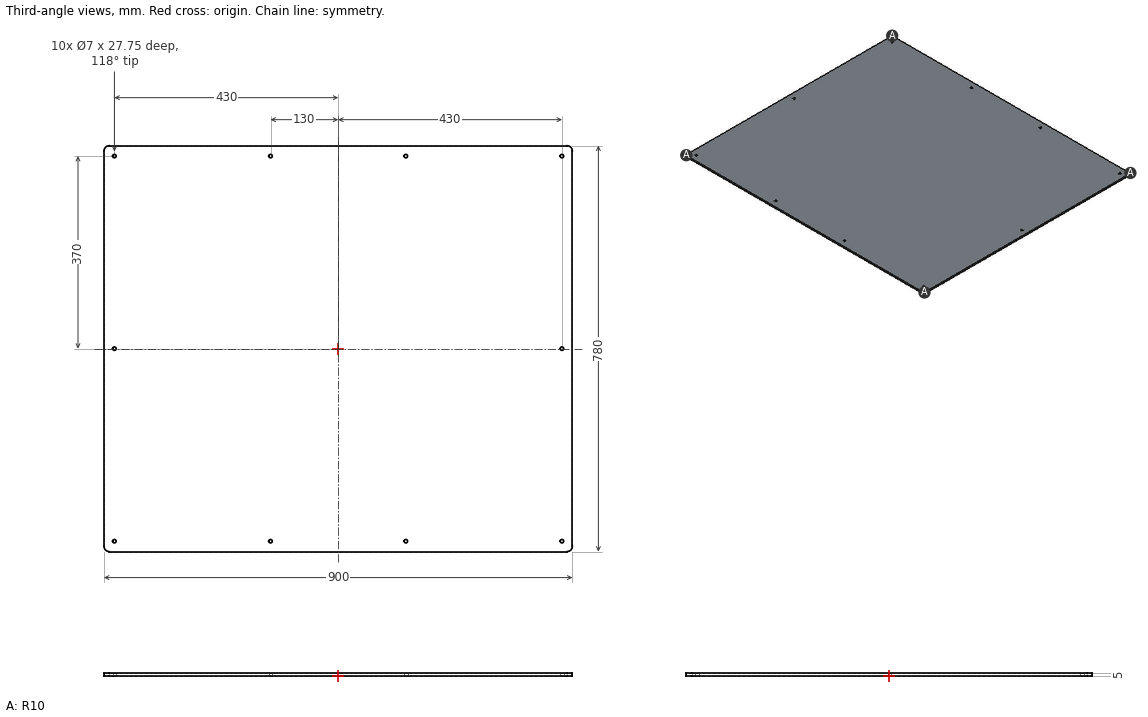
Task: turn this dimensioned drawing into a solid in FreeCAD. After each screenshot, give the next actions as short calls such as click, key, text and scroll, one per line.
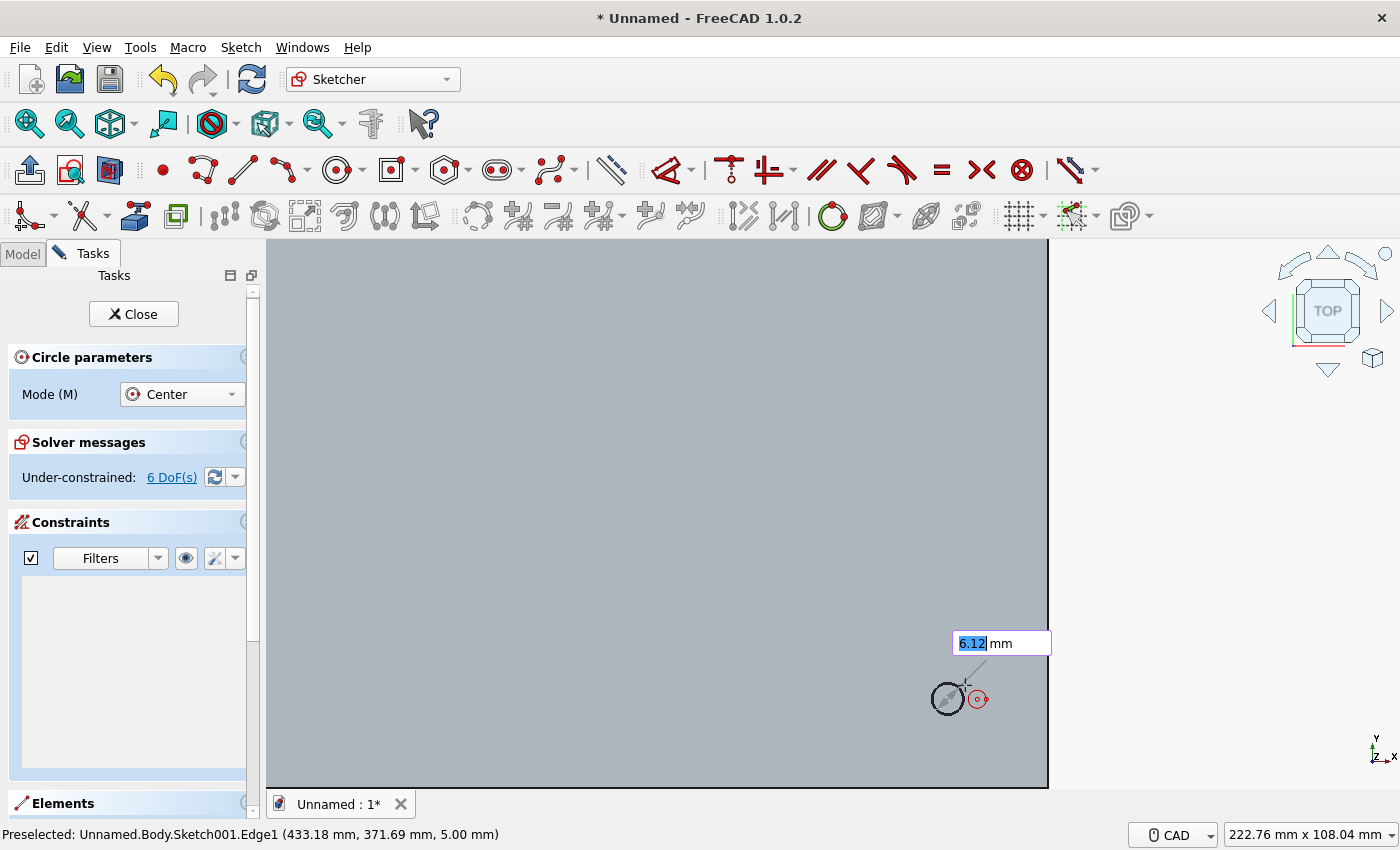
click(959, 673)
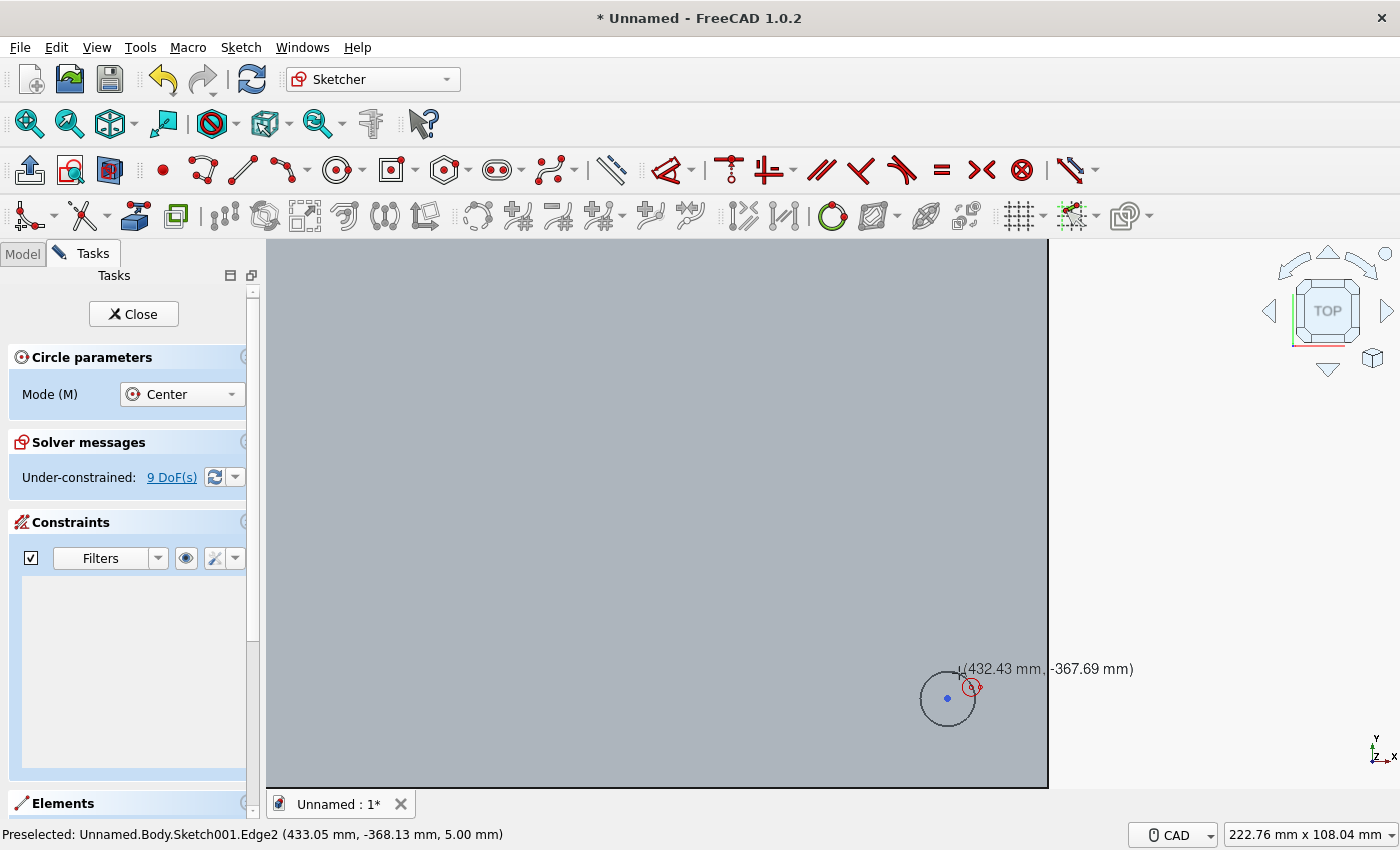
scroll(965, 685, down, 12)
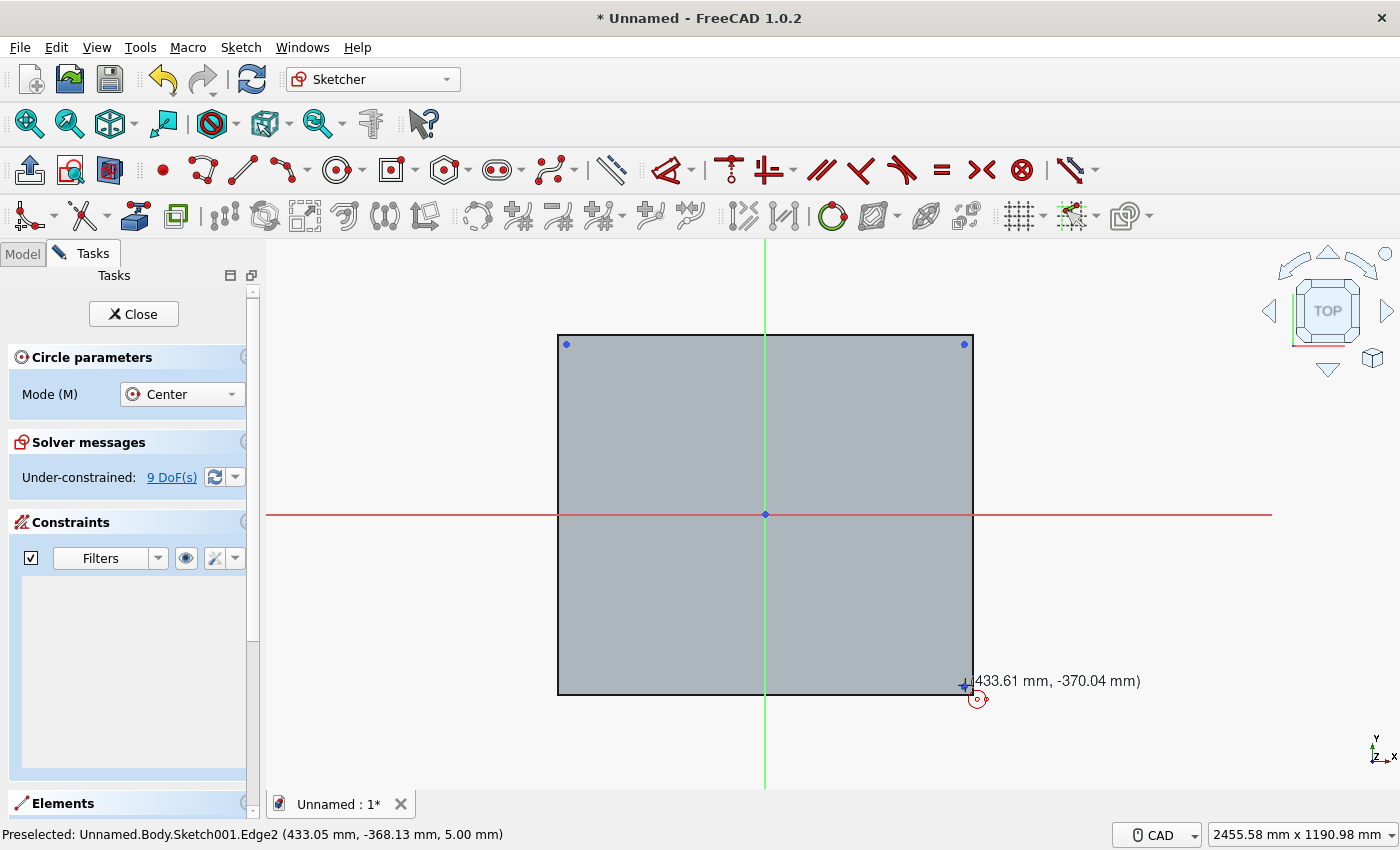
scroll(567, 686, up, 14)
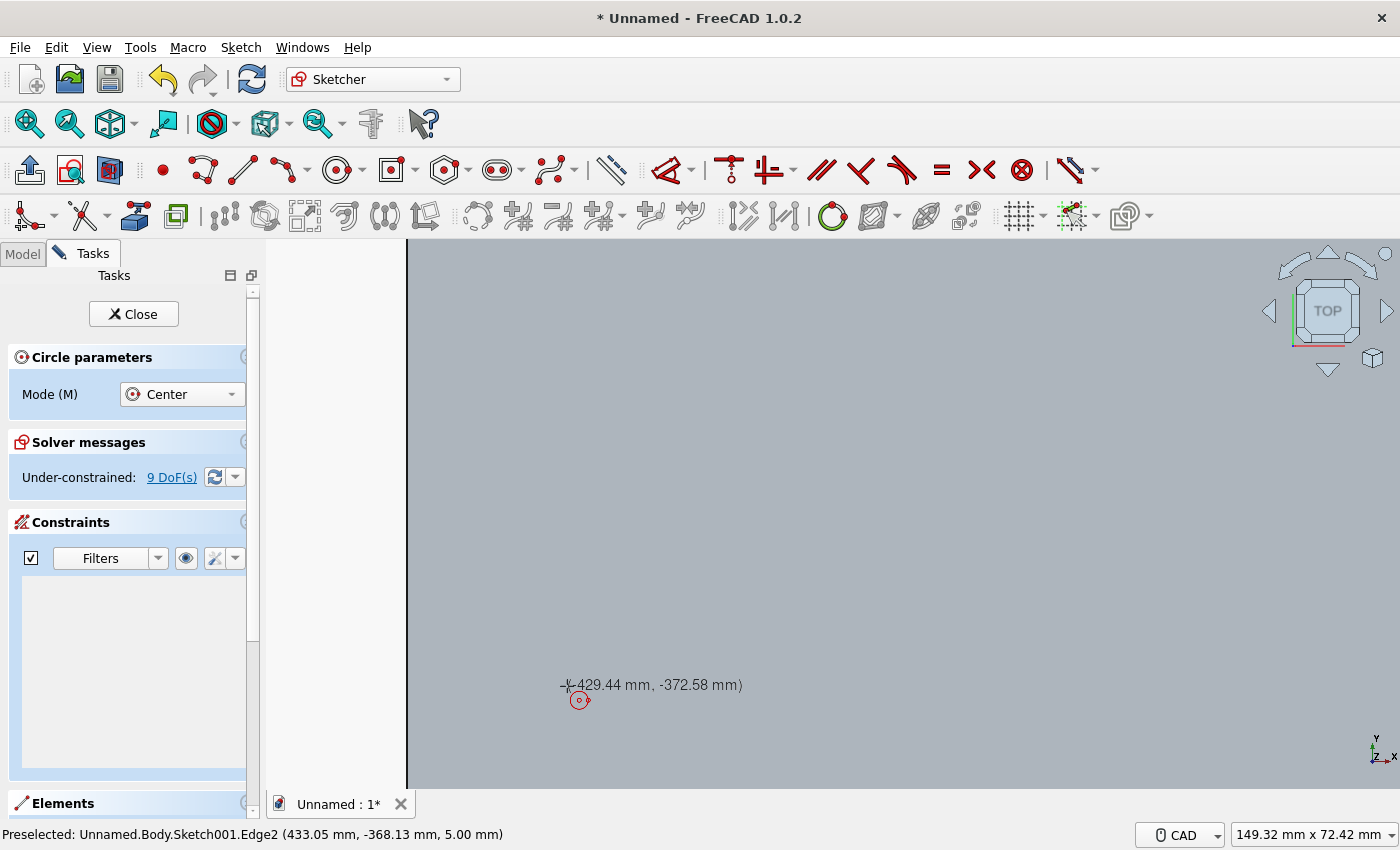
scroll(566, 686, down, 14)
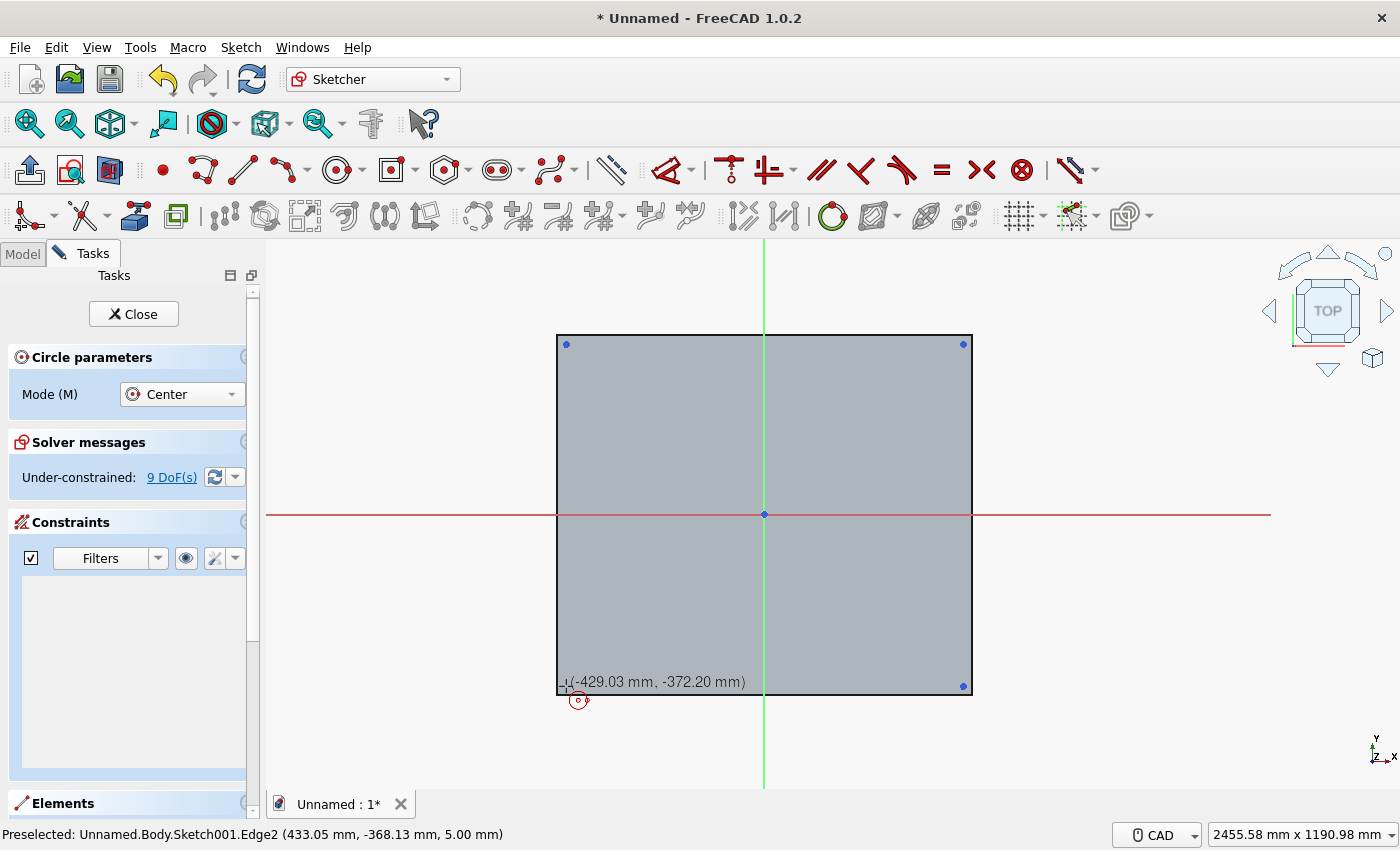
click(566, 686)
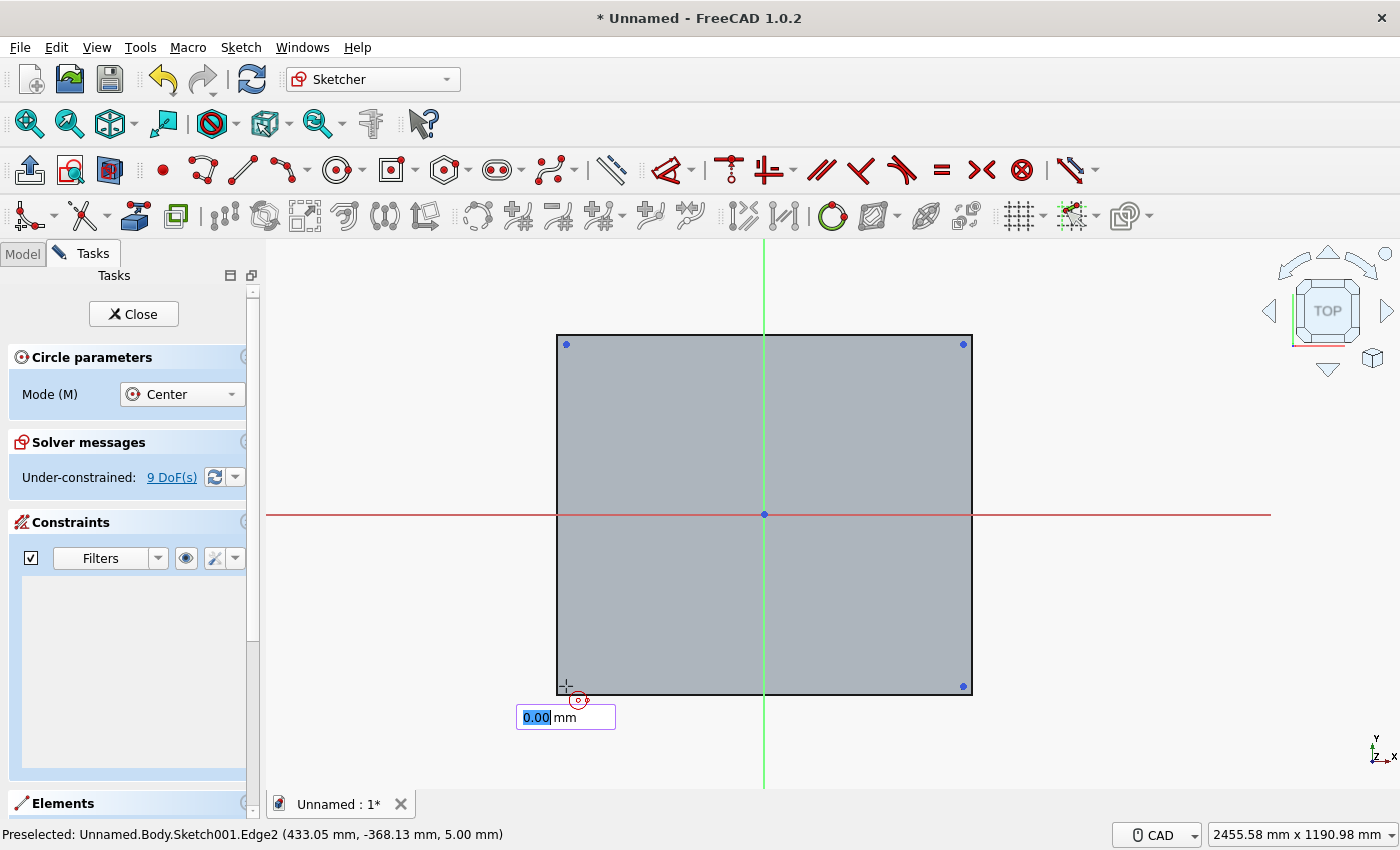
scroll(567, 685, up, 12)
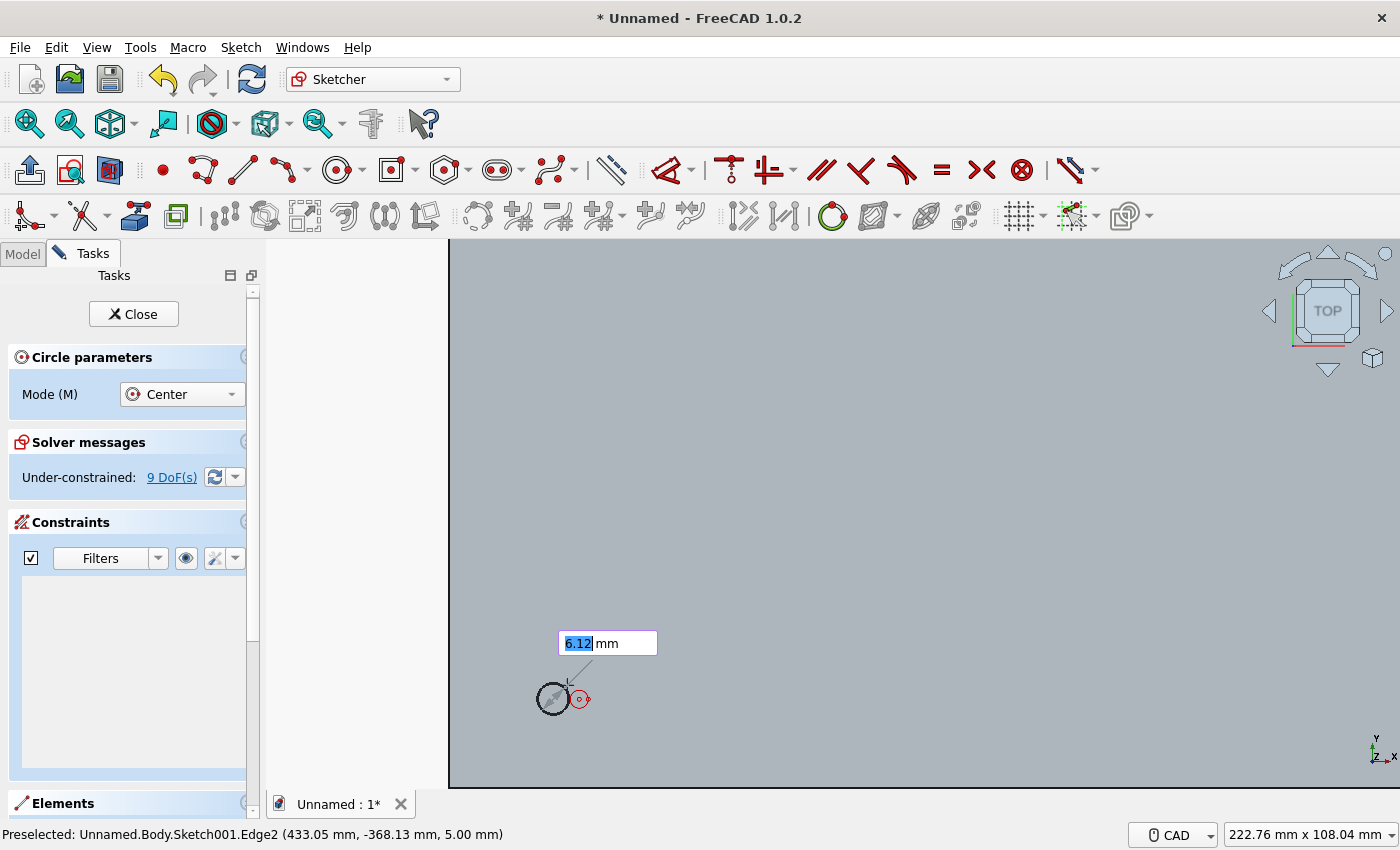
click(564, 673)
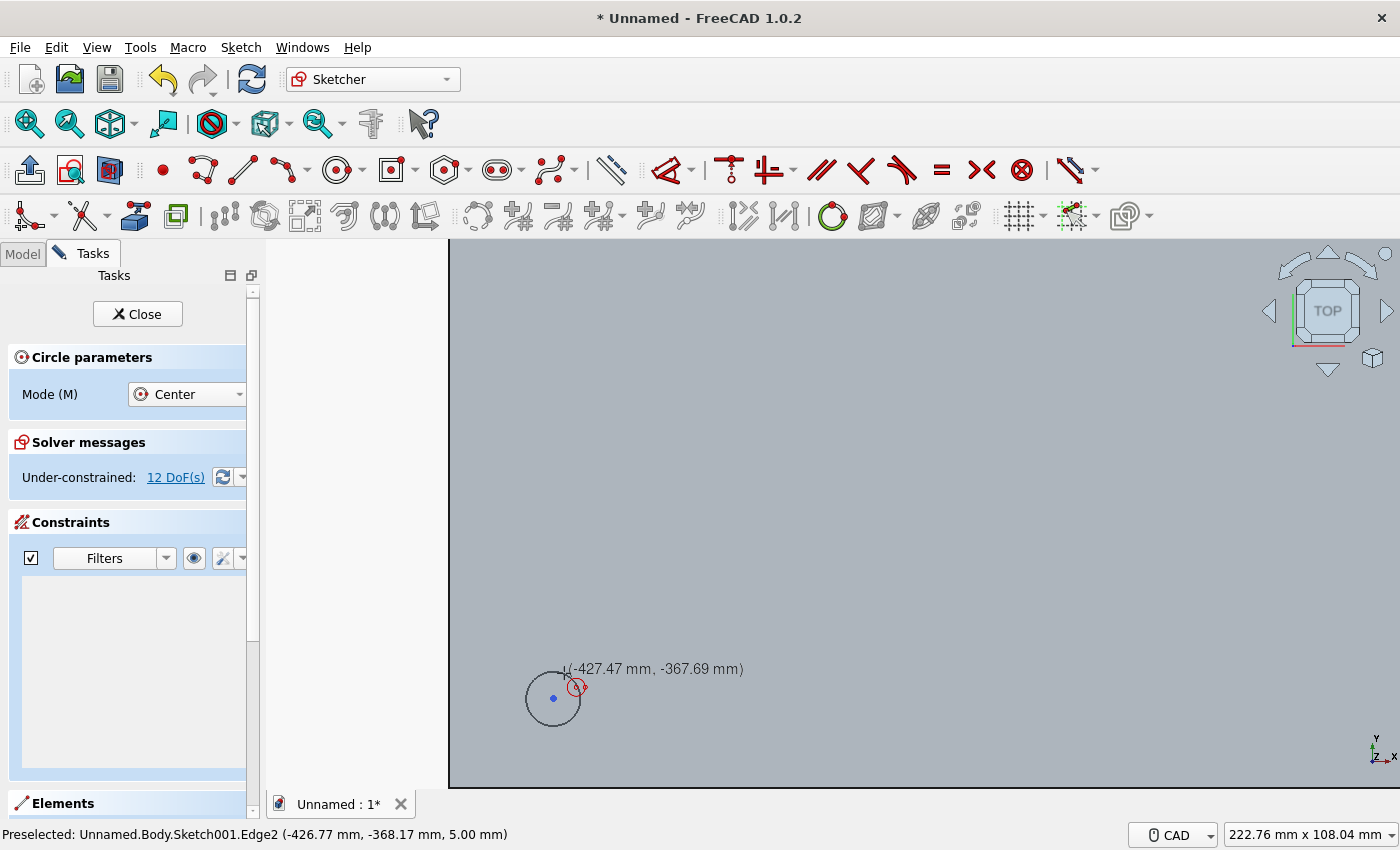
scroll(567, 685, down, 12)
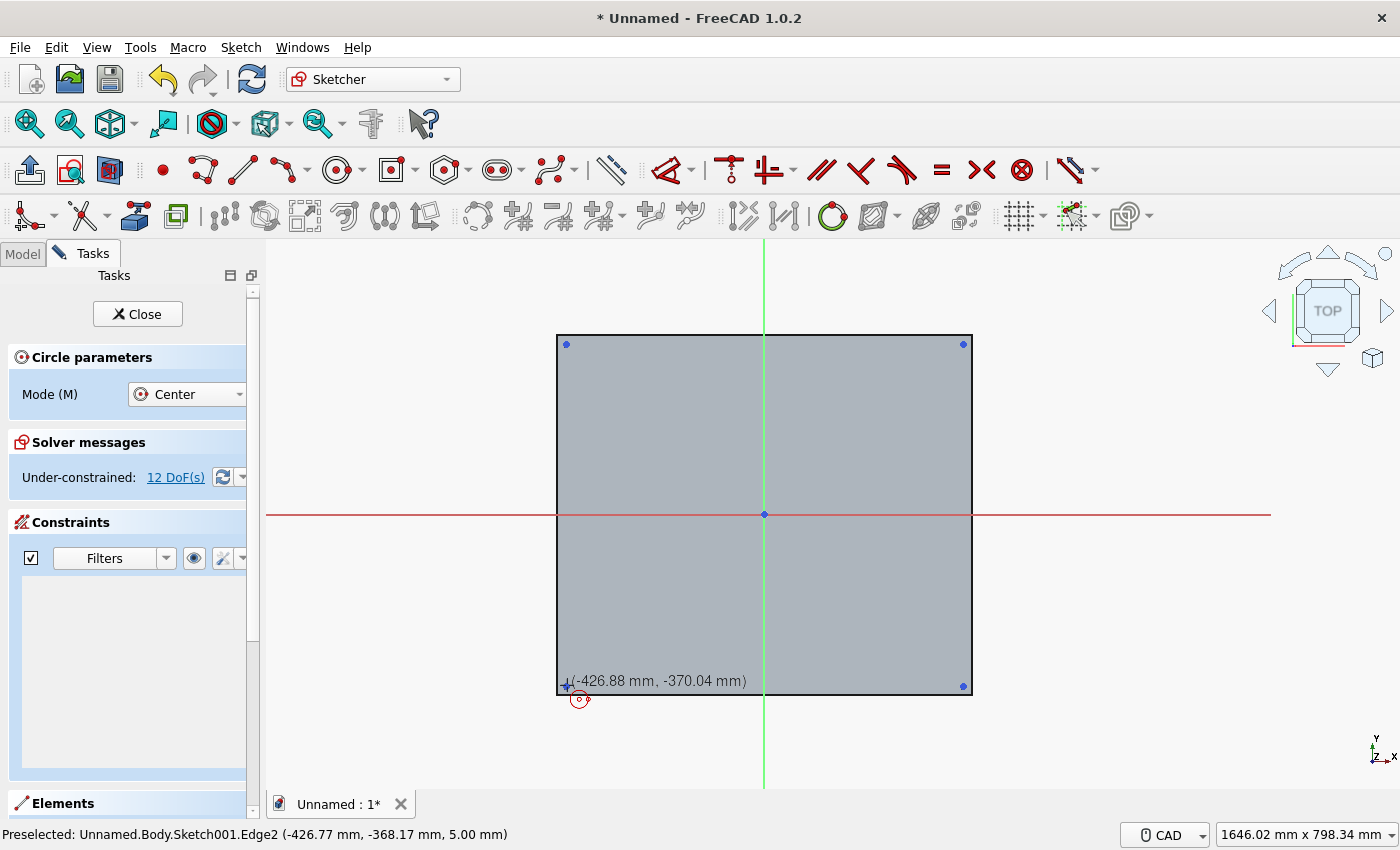
scroll(566, 515, up, 14)